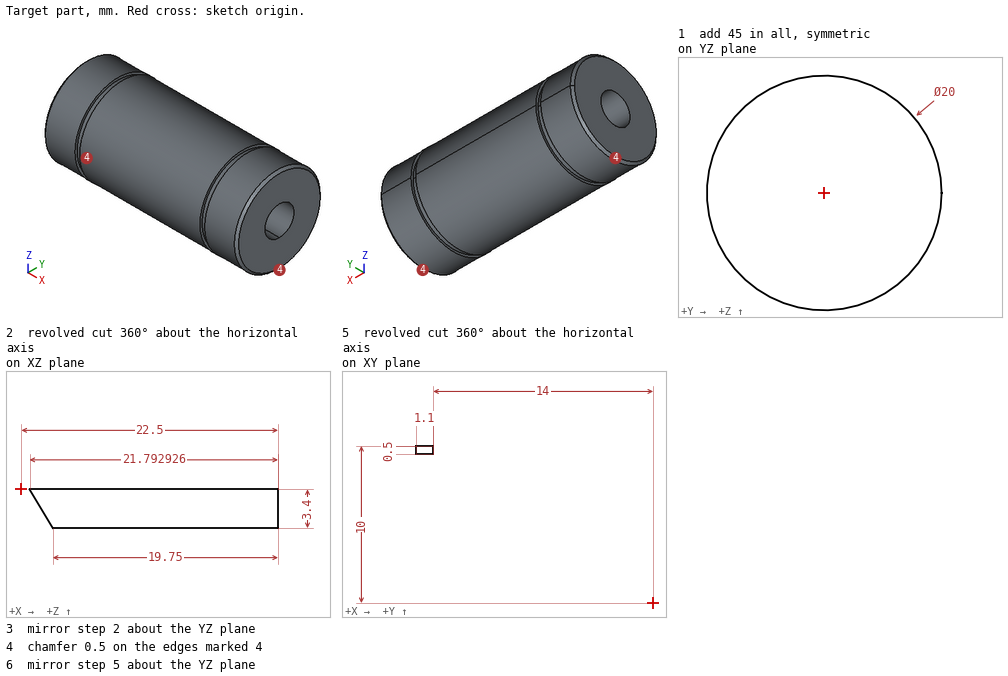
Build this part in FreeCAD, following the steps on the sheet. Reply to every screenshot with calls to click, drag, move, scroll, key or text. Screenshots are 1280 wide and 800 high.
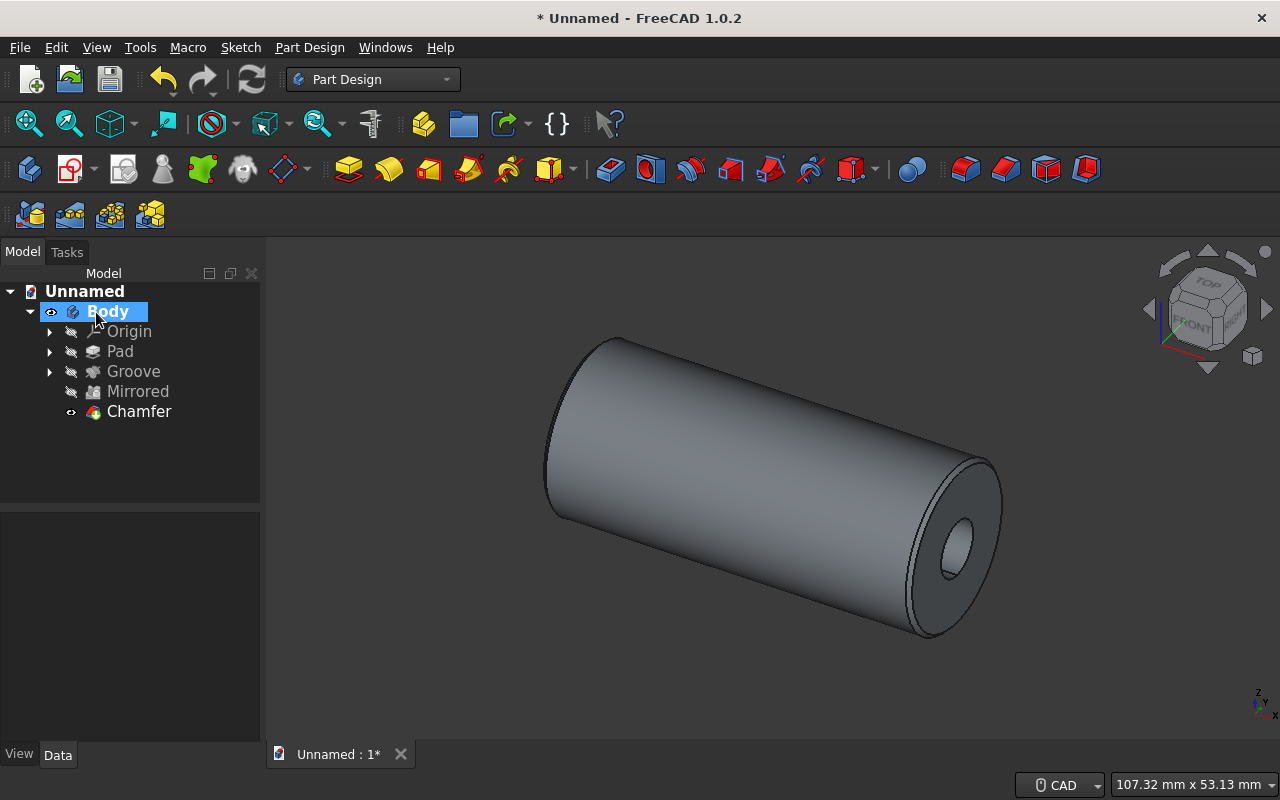
click(70, 170)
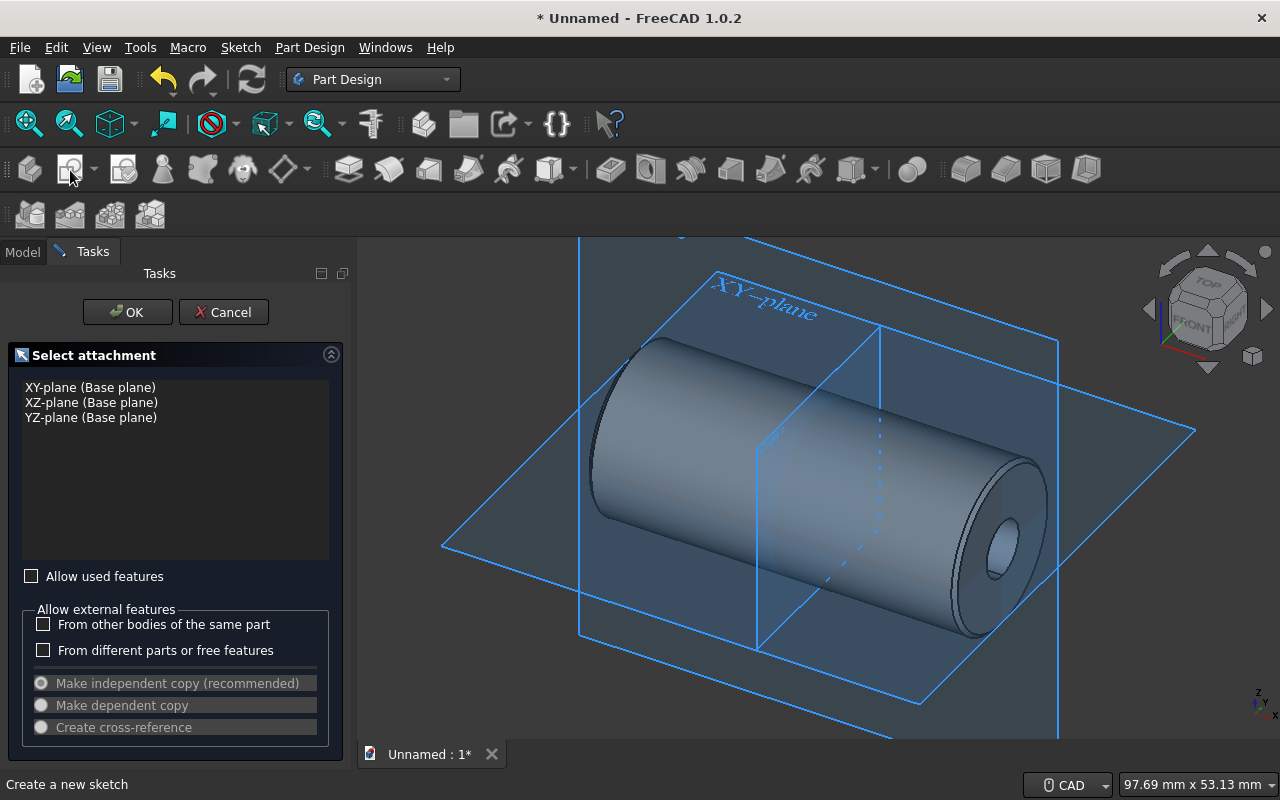
click(82, 388)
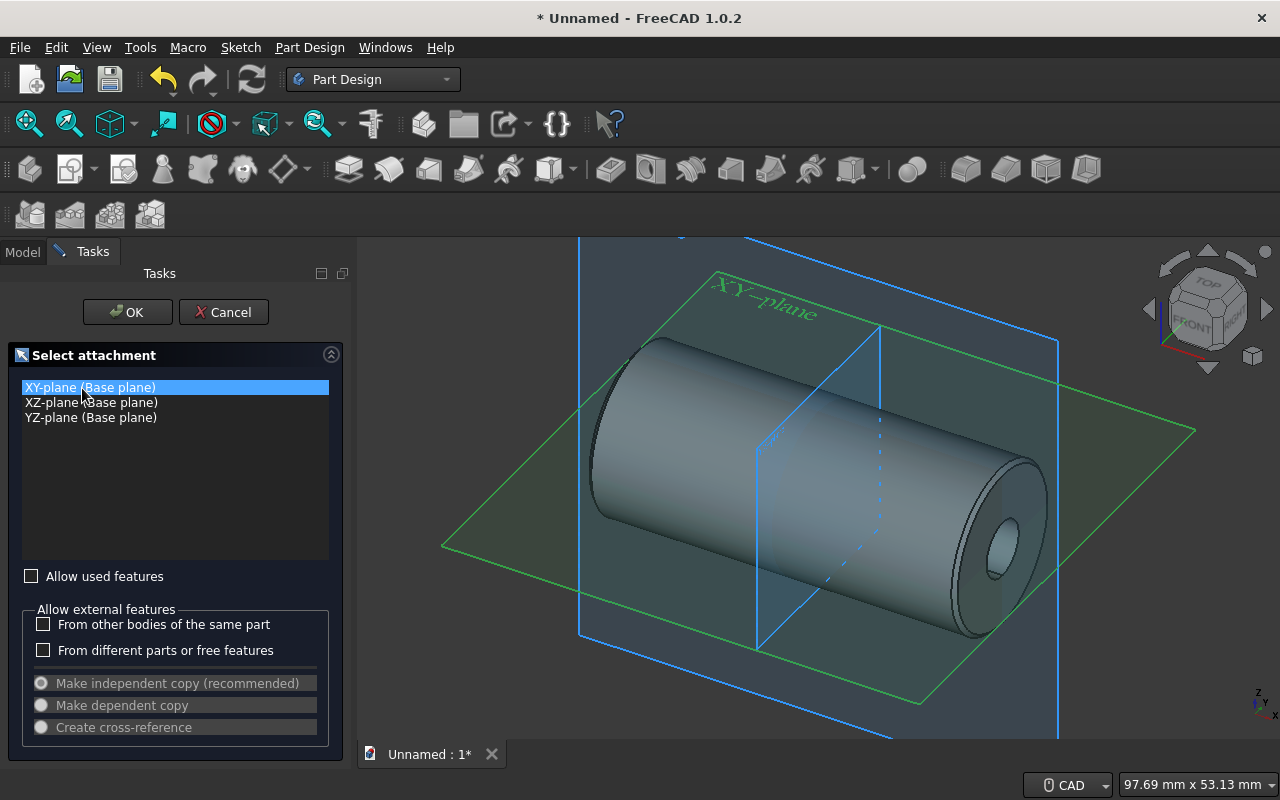
click(128, 312)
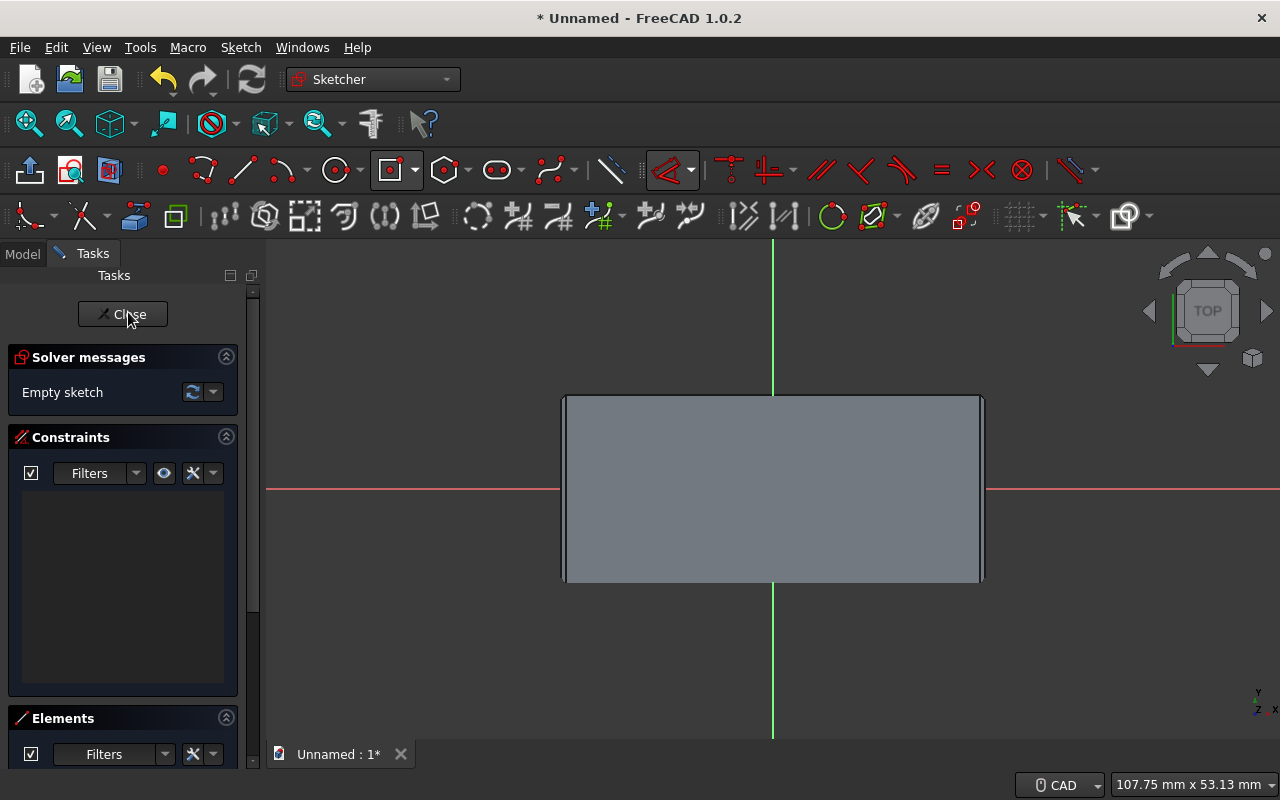
key(q)
key(s)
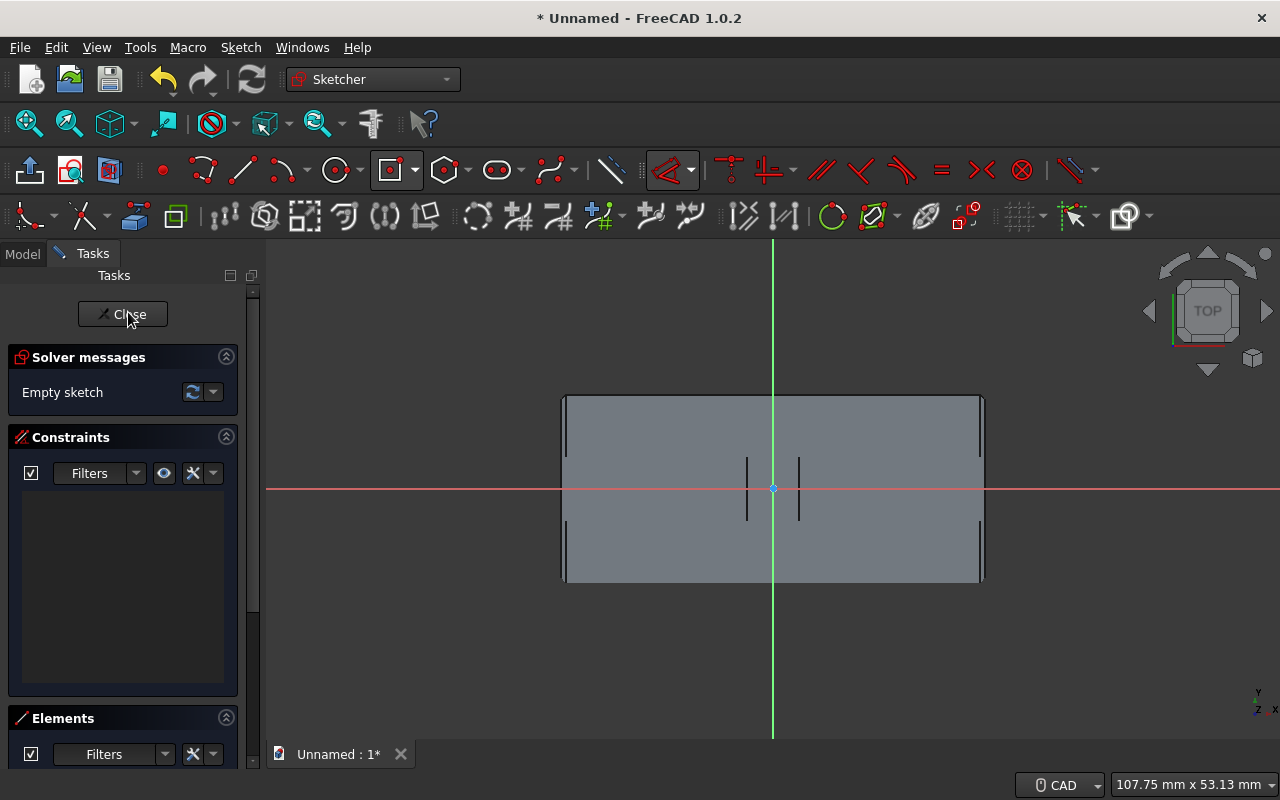
scroll(632, 392, up, 15)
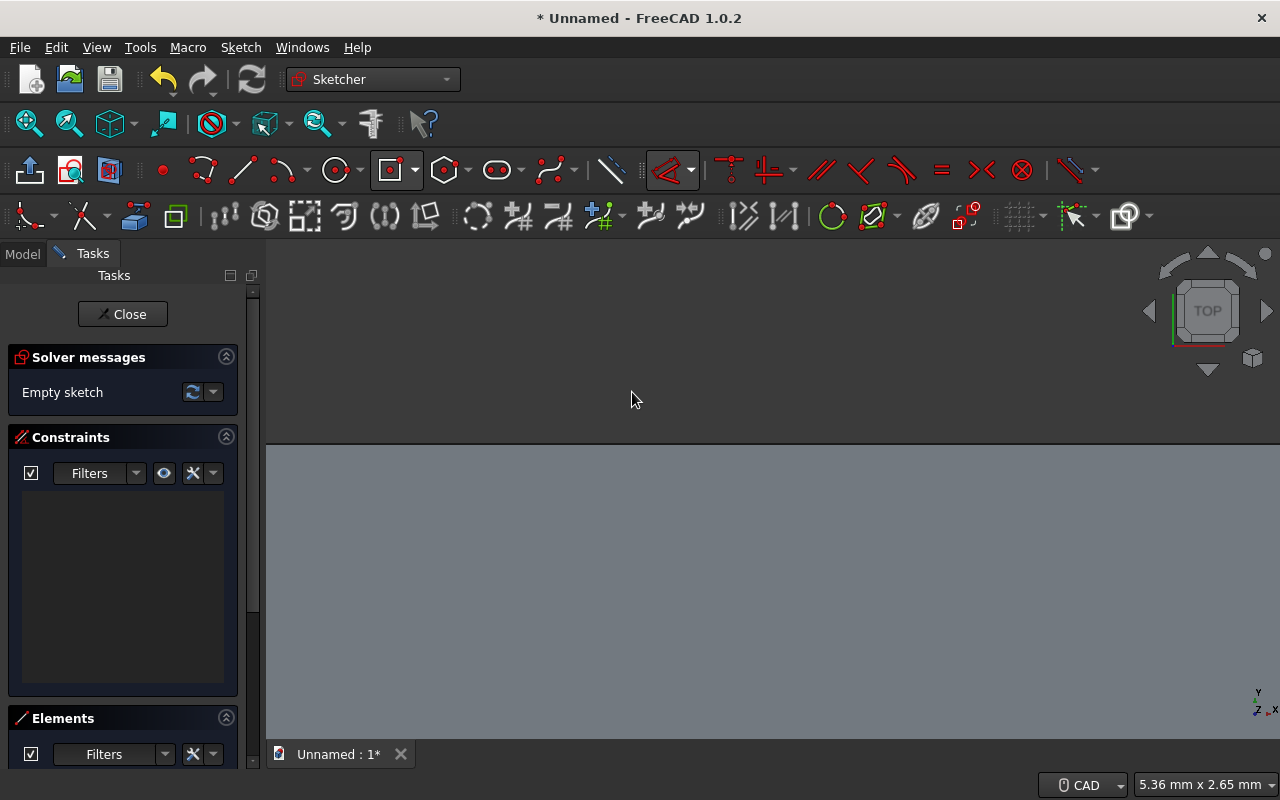
scroll(708, 493, up, 5)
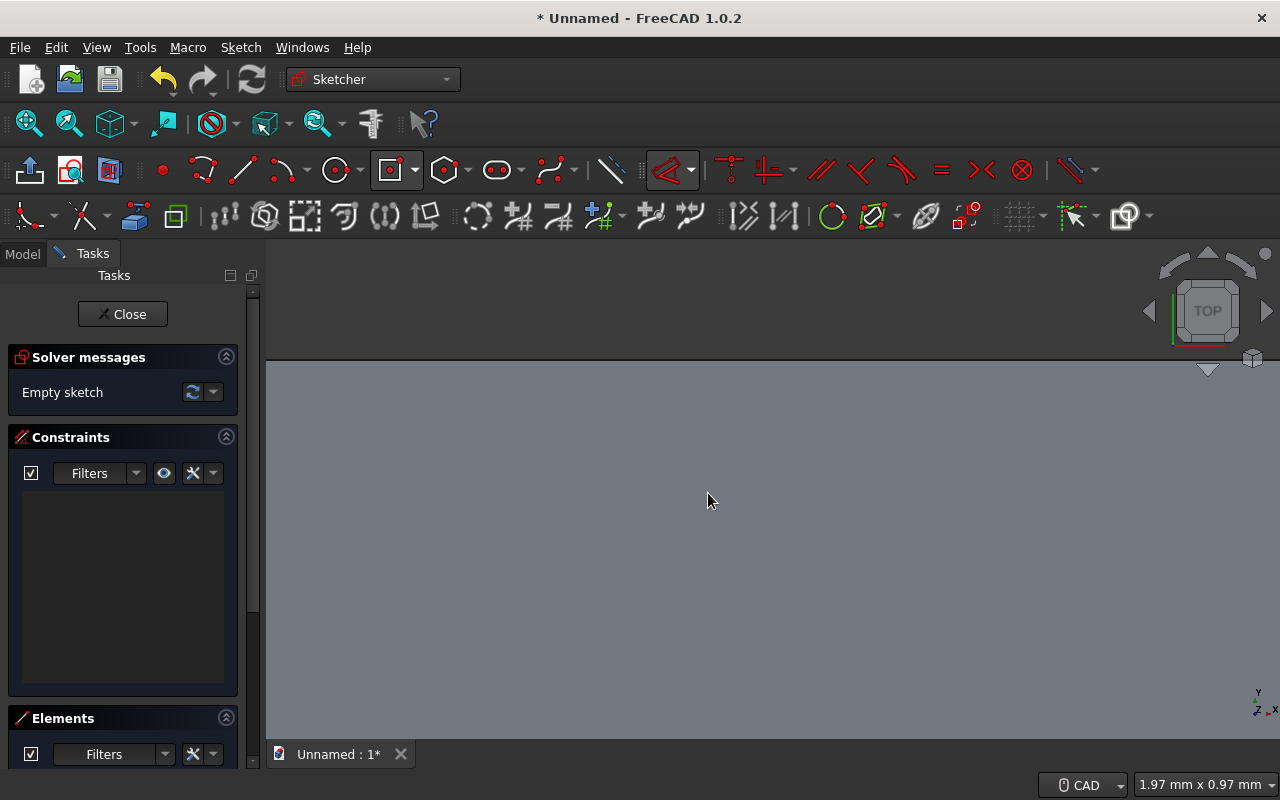
click(418, 170)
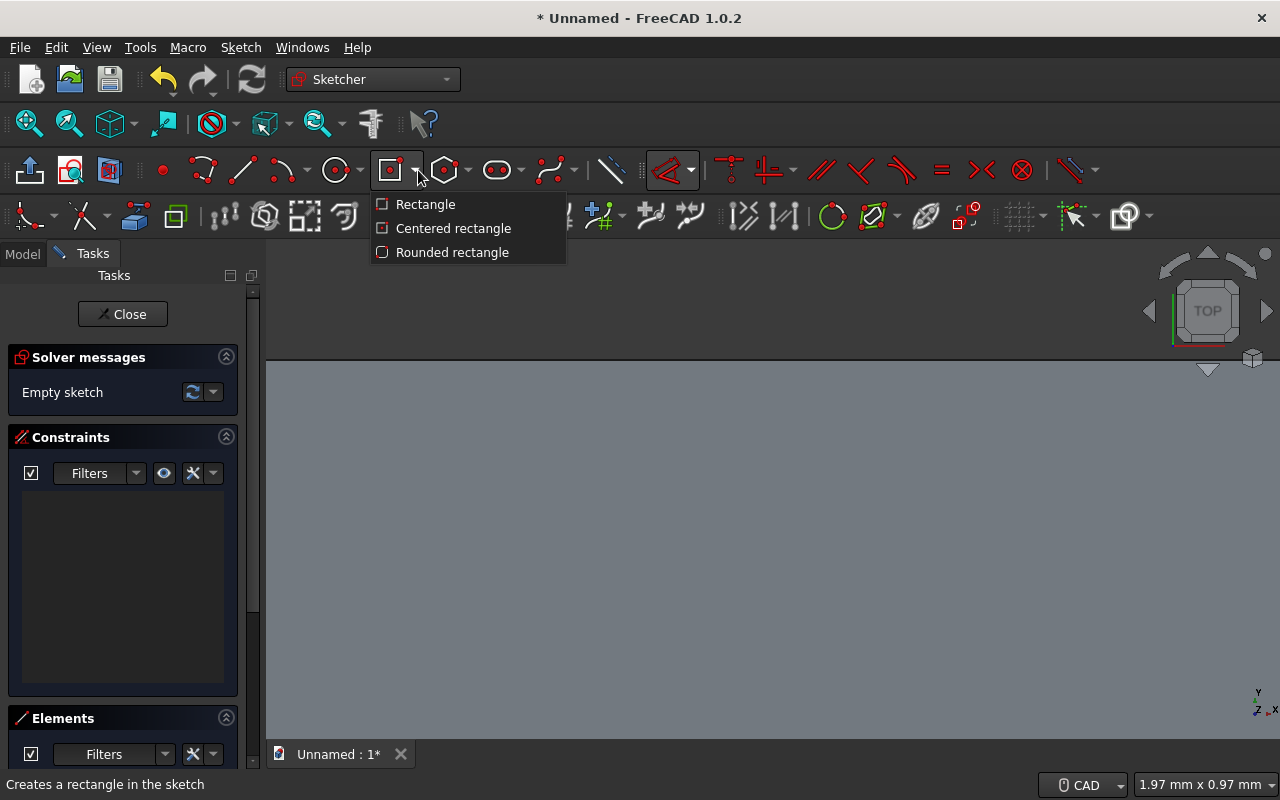
click(468, 204)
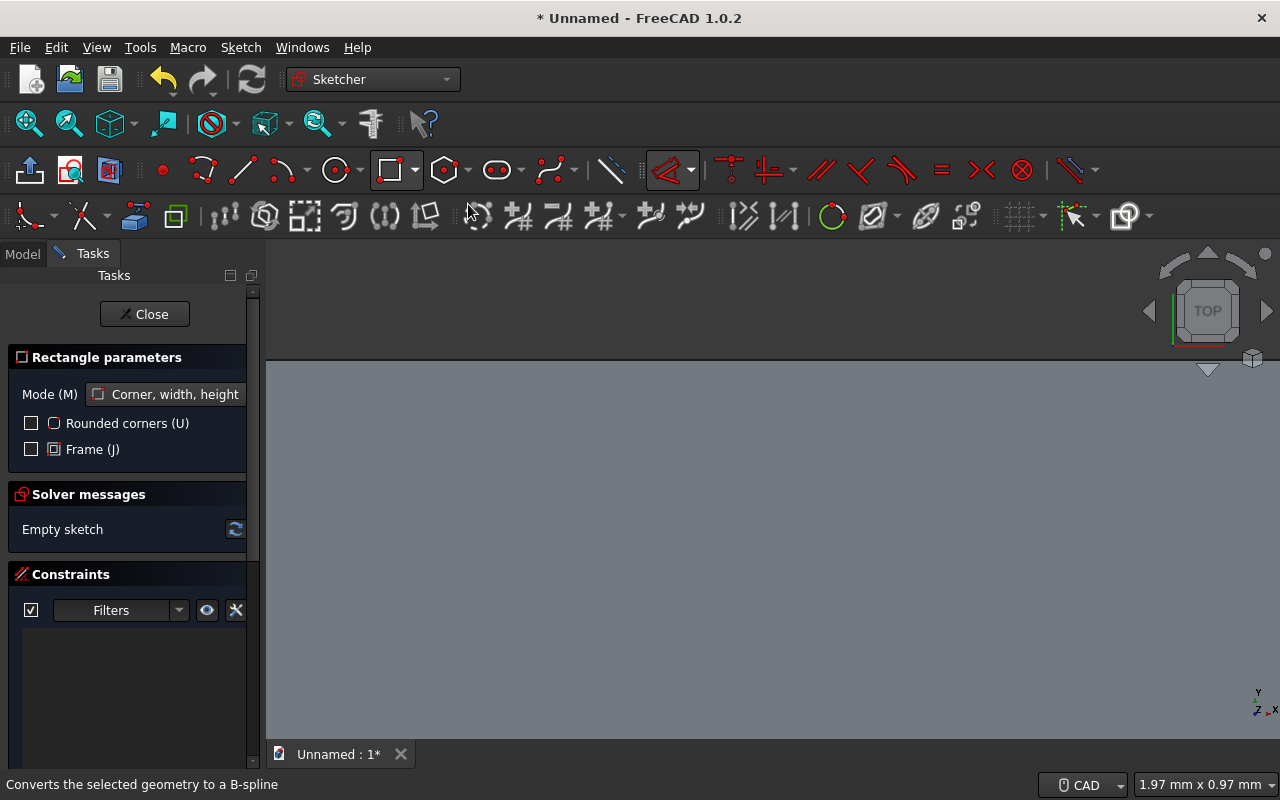
click(422, 360)
move(987, 616)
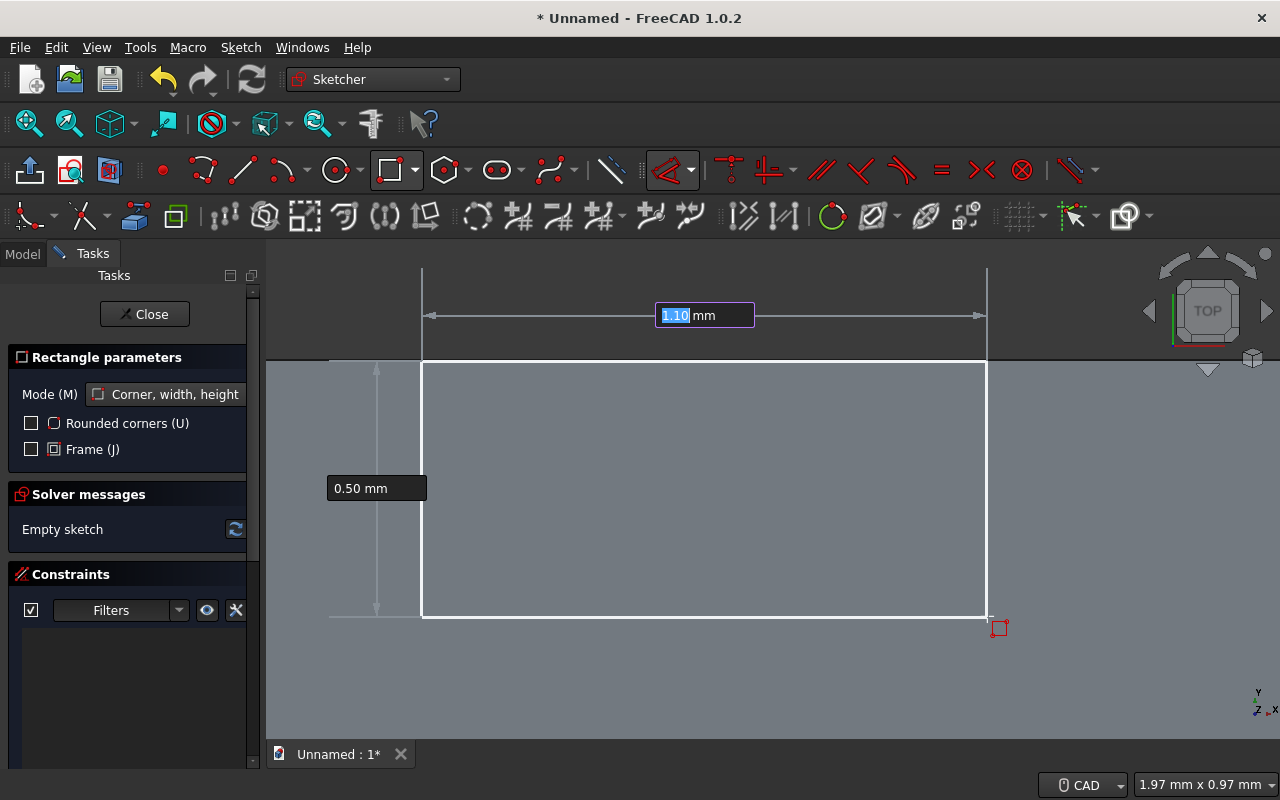
text(1.1)
key(Tab)
text(0.5)
key(Return)
key(Escape)